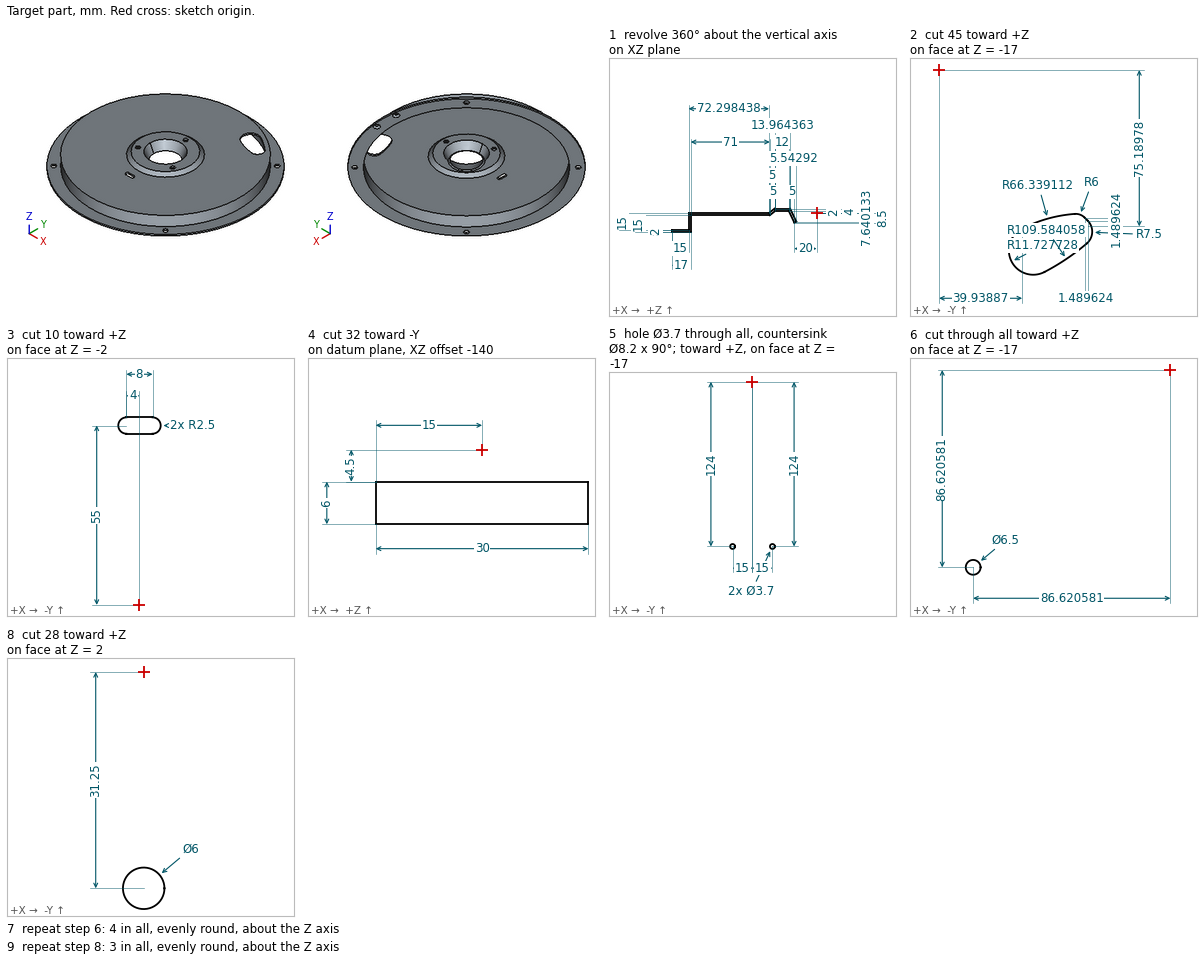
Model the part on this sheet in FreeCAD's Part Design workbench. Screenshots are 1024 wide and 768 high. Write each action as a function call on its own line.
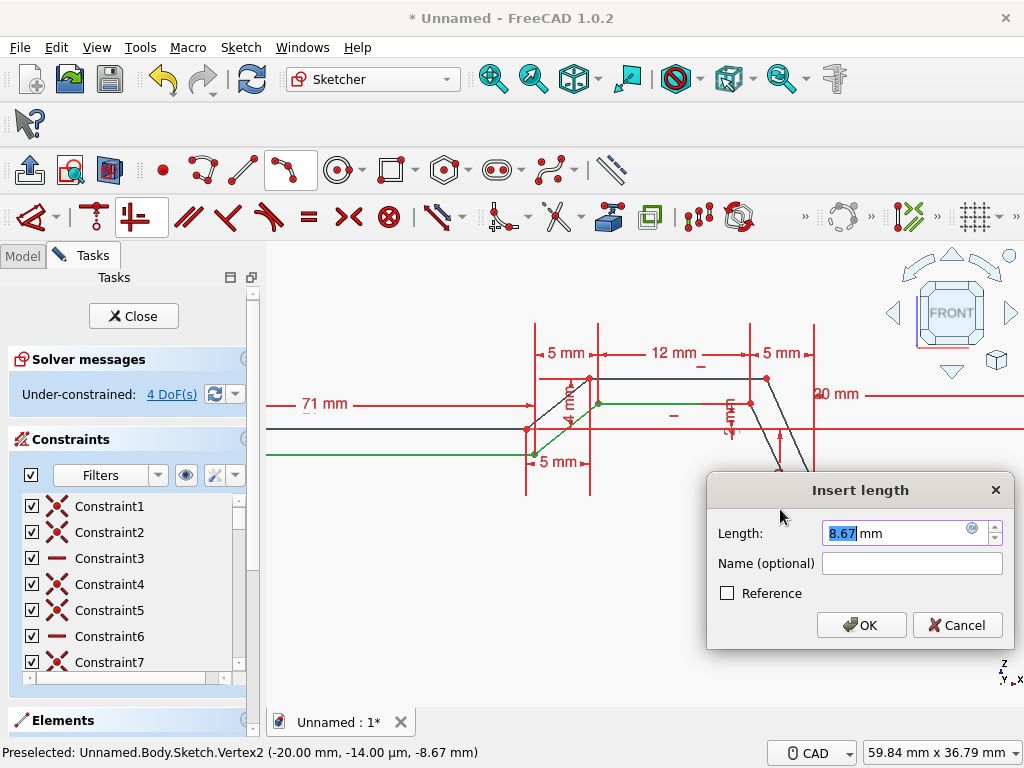
text(8.5)
key(Return)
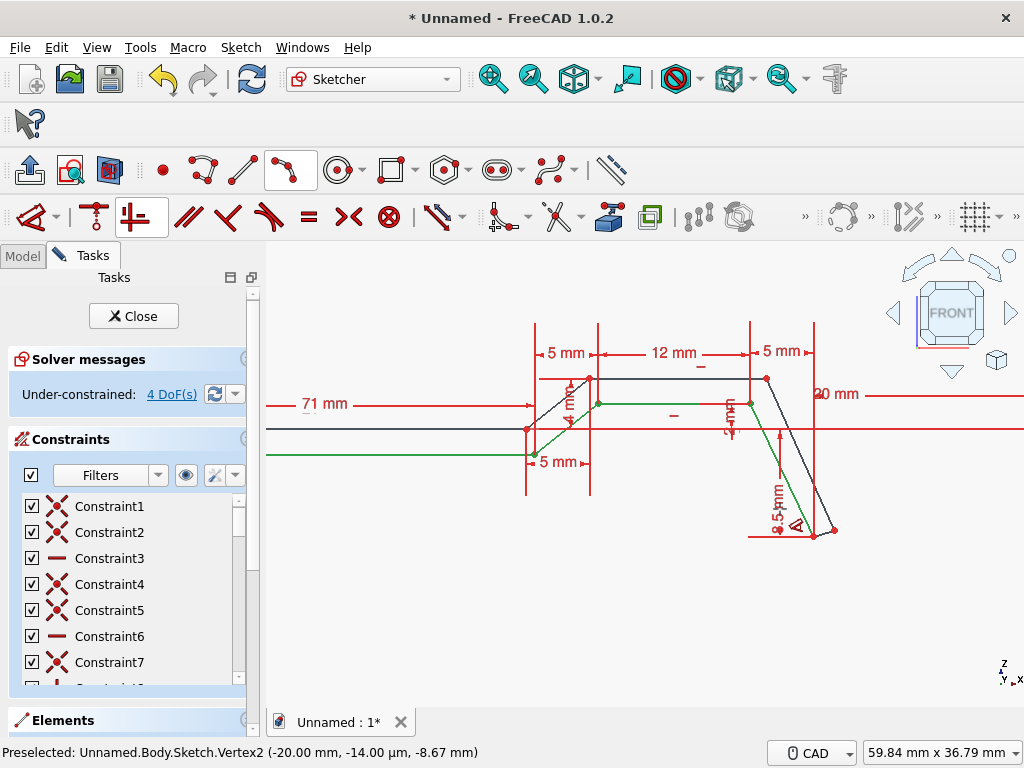
click(814, 485)
click(800, 565)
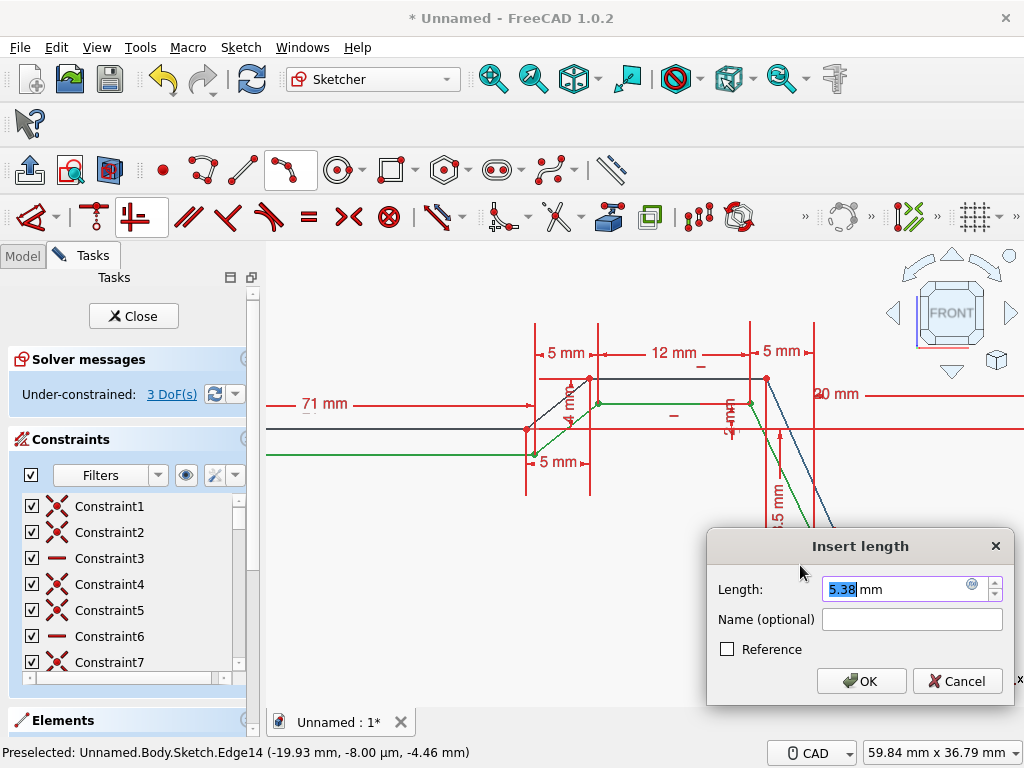
text(5.54292)
key(Return)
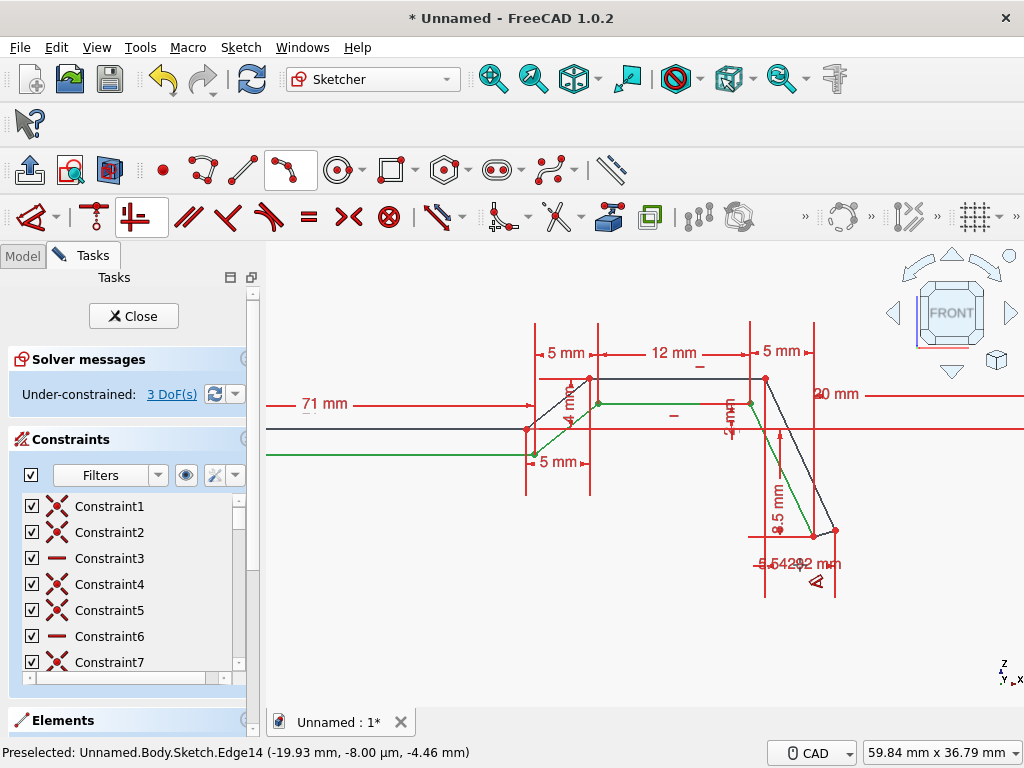
click(343, 429)
click(410, 395)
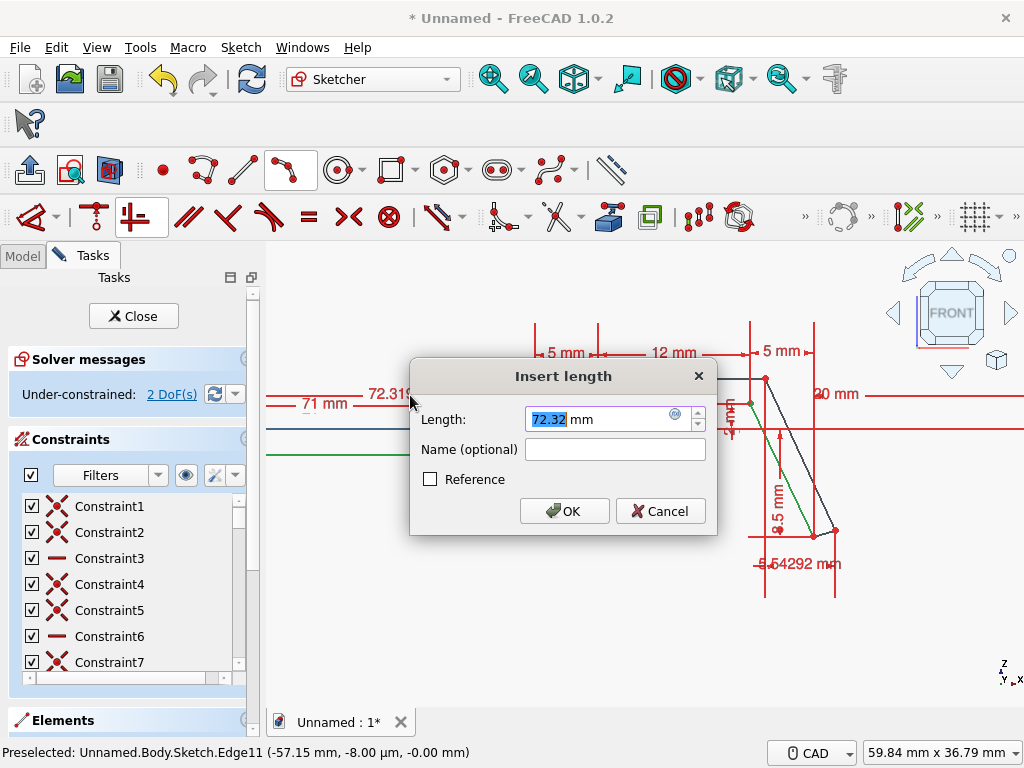
text(72.298438)
key(Return)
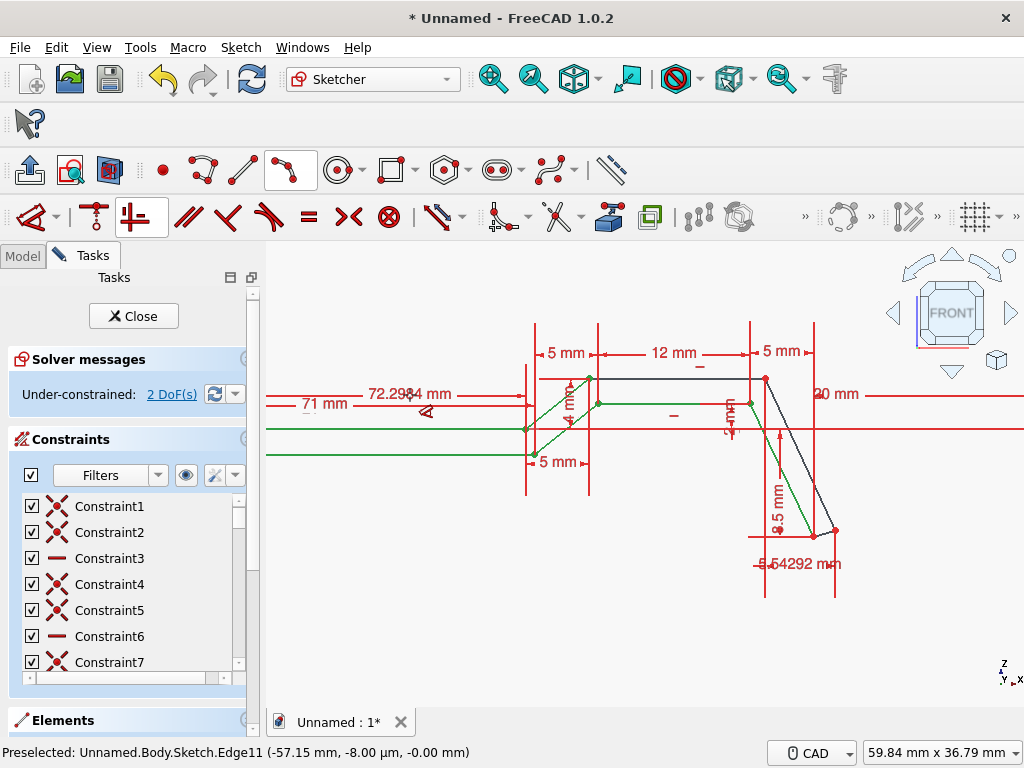
click(642, 379)
click(677, 321)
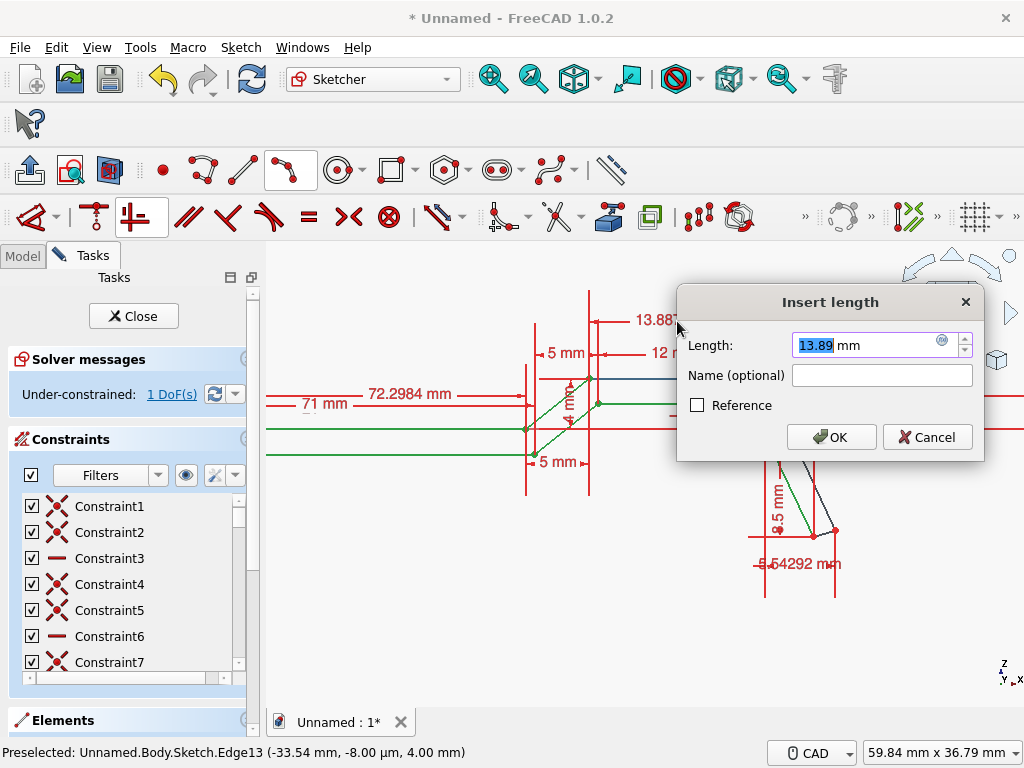
text(13.964363)
key(Return)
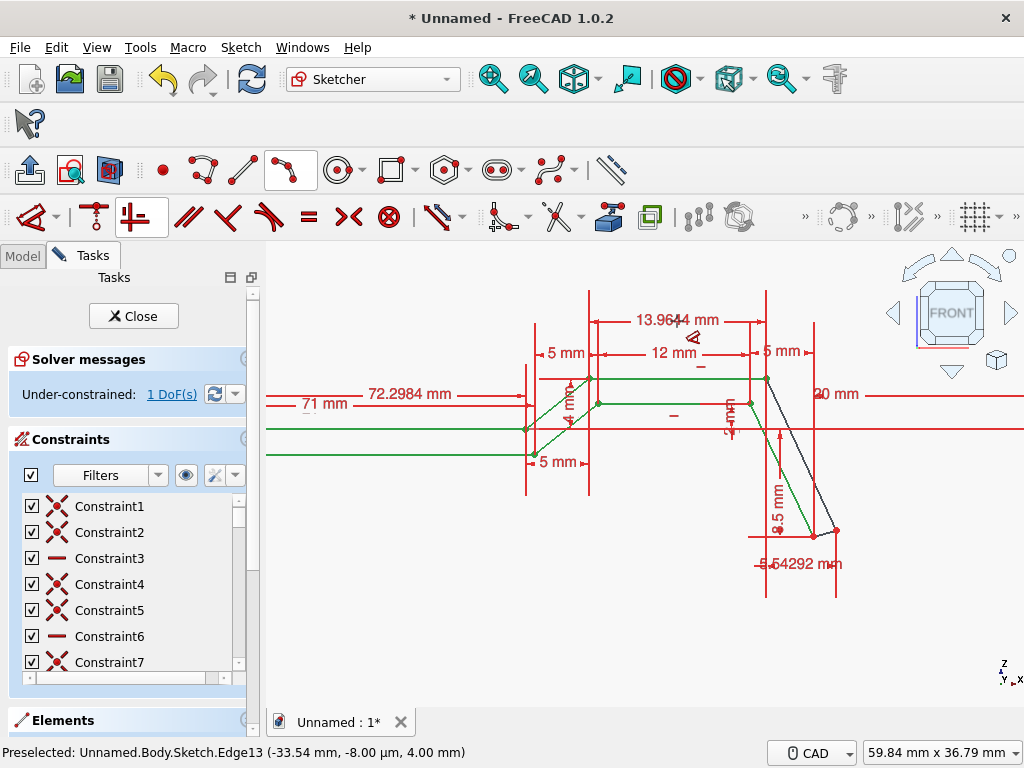
click(836, 531)
click(754, 480)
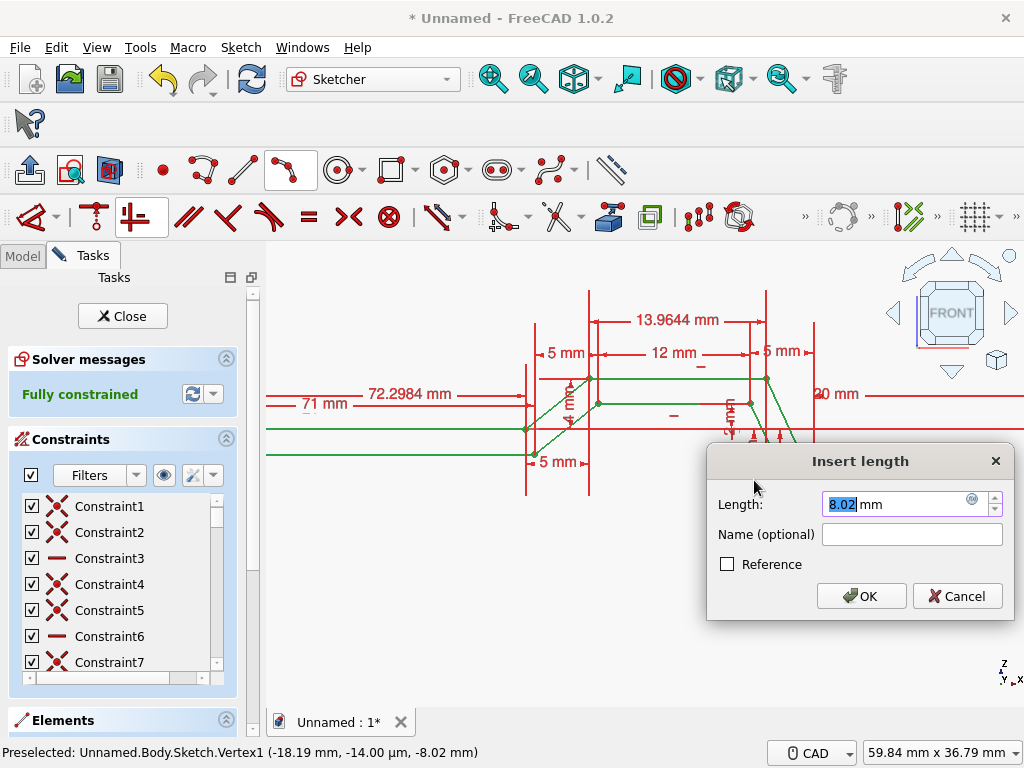
text(7.640133)
key(Return)
key(Escape)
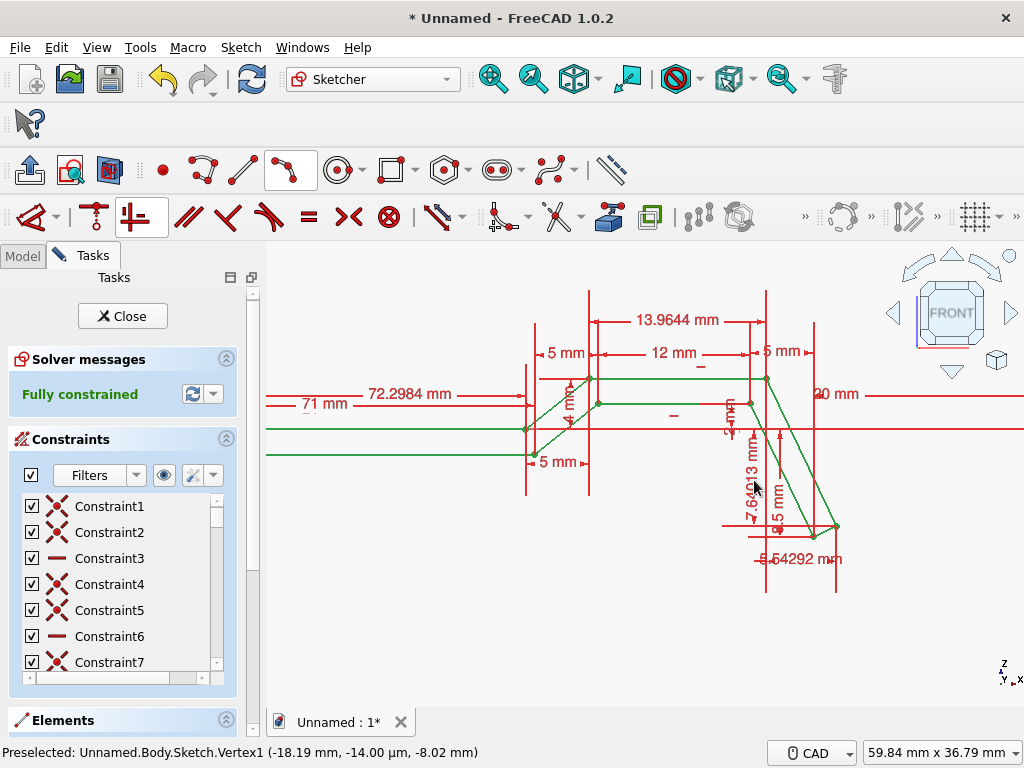
click(123, 316)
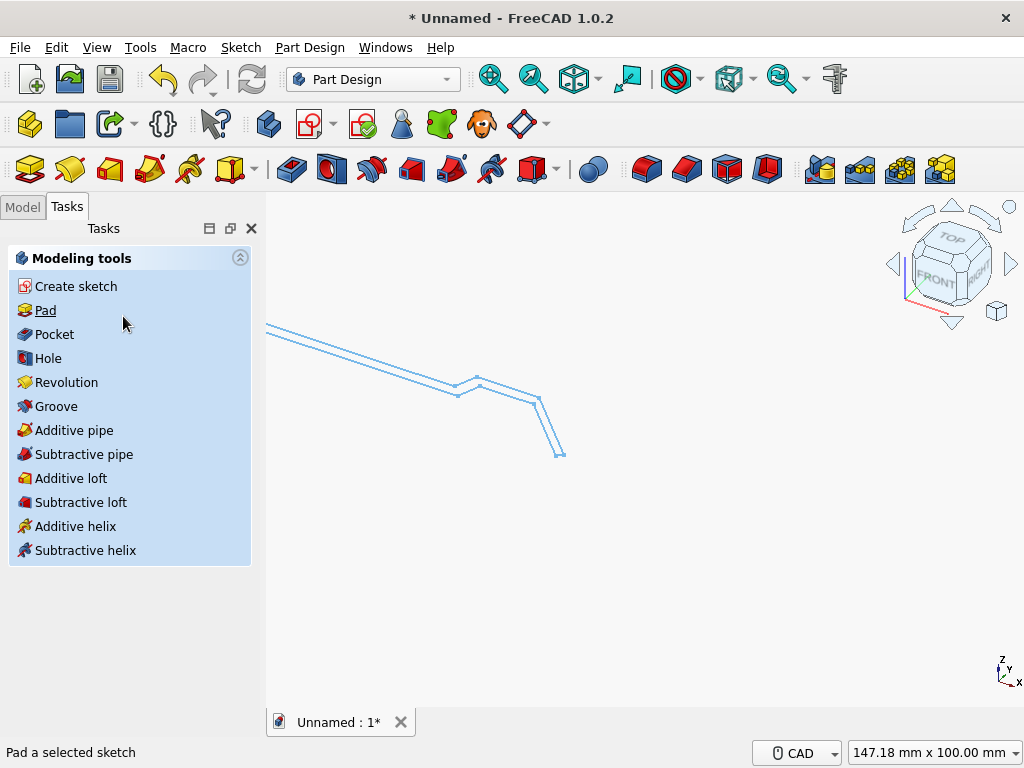
click(70, 170)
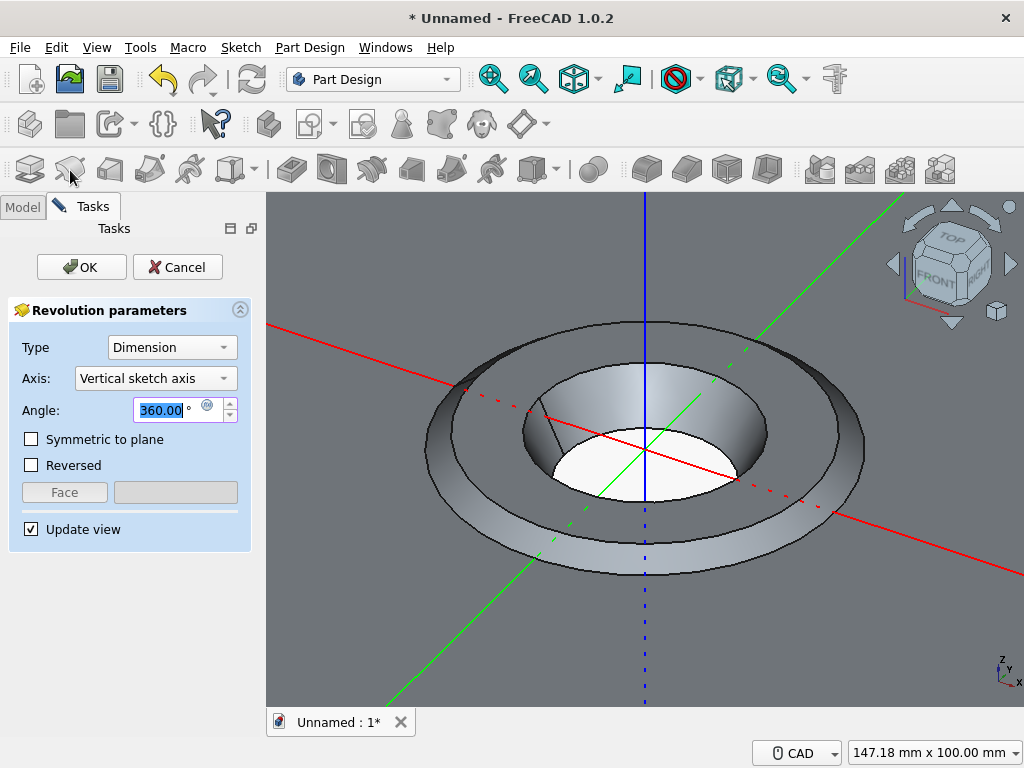
click(82, 267)